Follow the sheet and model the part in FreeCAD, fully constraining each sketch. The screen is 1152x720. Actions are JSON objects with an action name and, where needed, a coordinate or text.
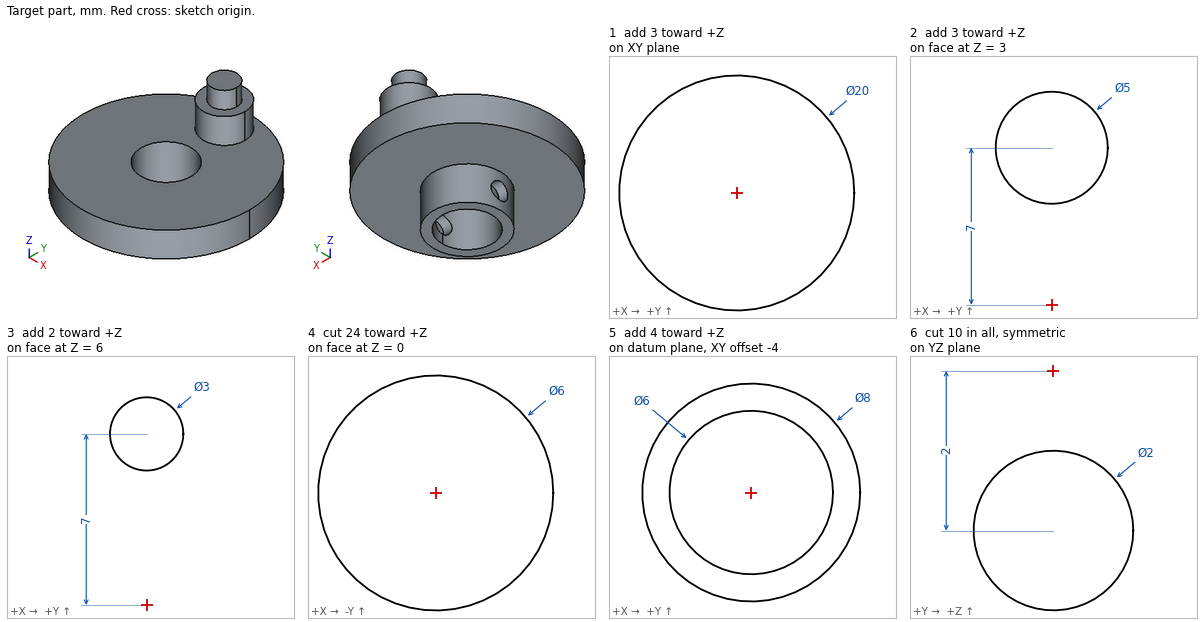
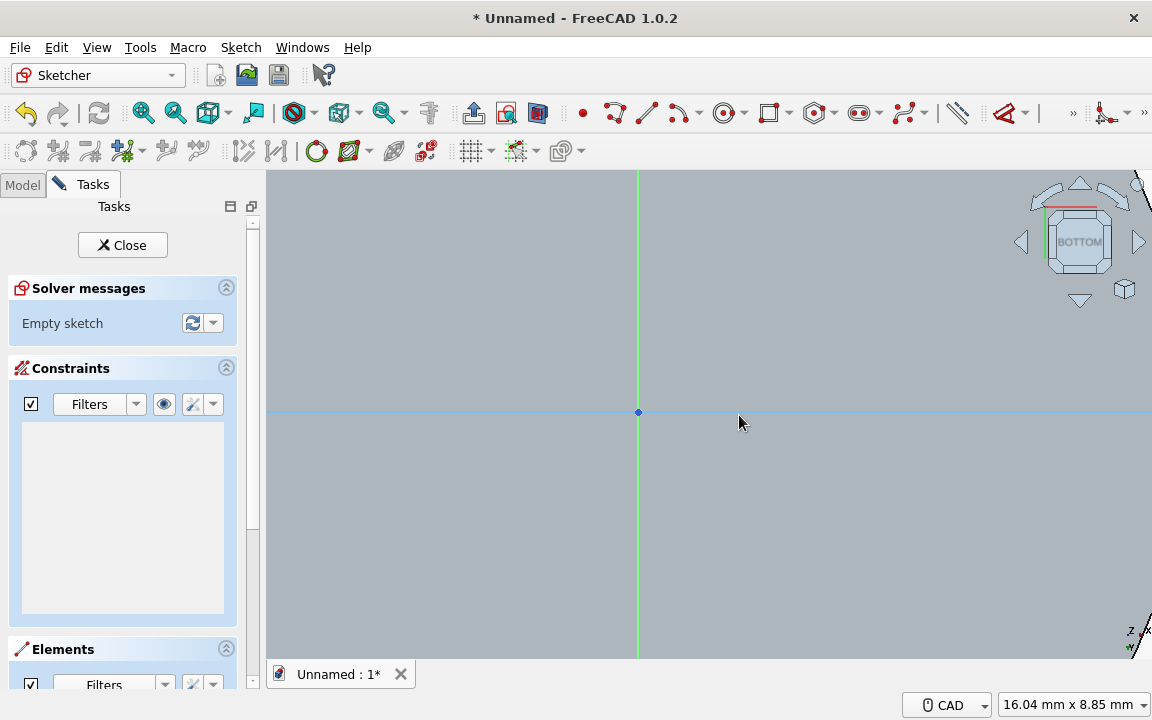
{"action": "key", "text": "g c"}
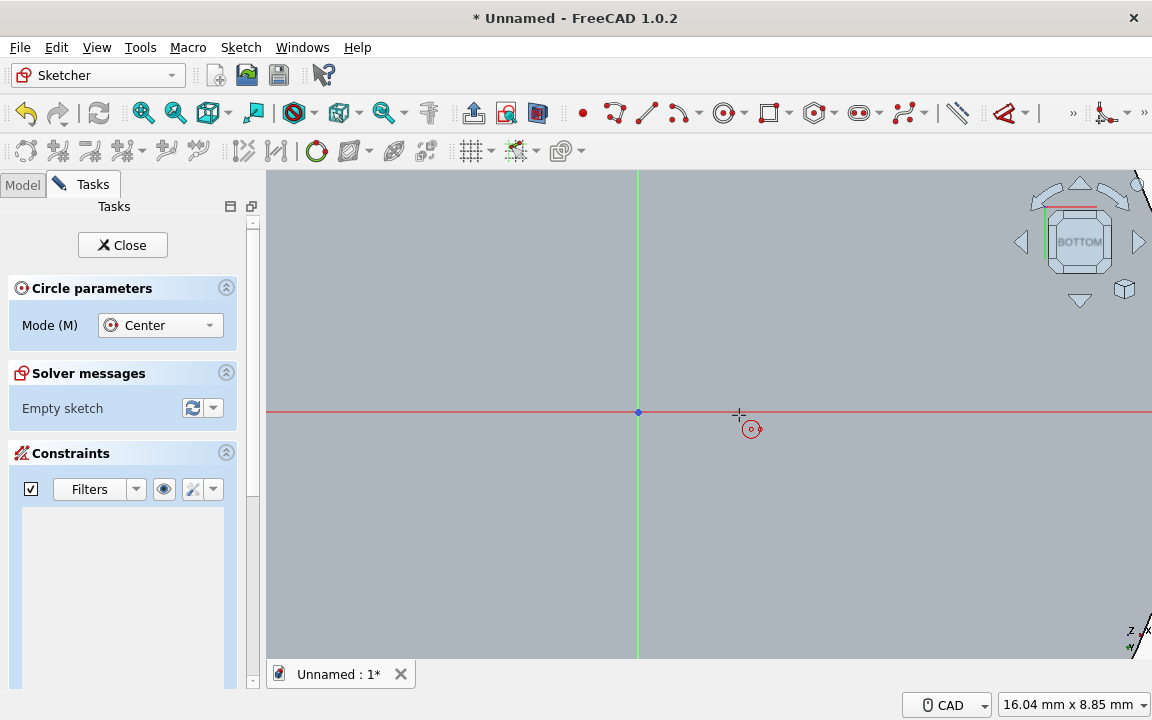
{"action": "left_click", "coordinate": [638, 412]}
{"action": "left_click", "coordinate": [755, 295]}
{"action": "key", "text": "Escape"}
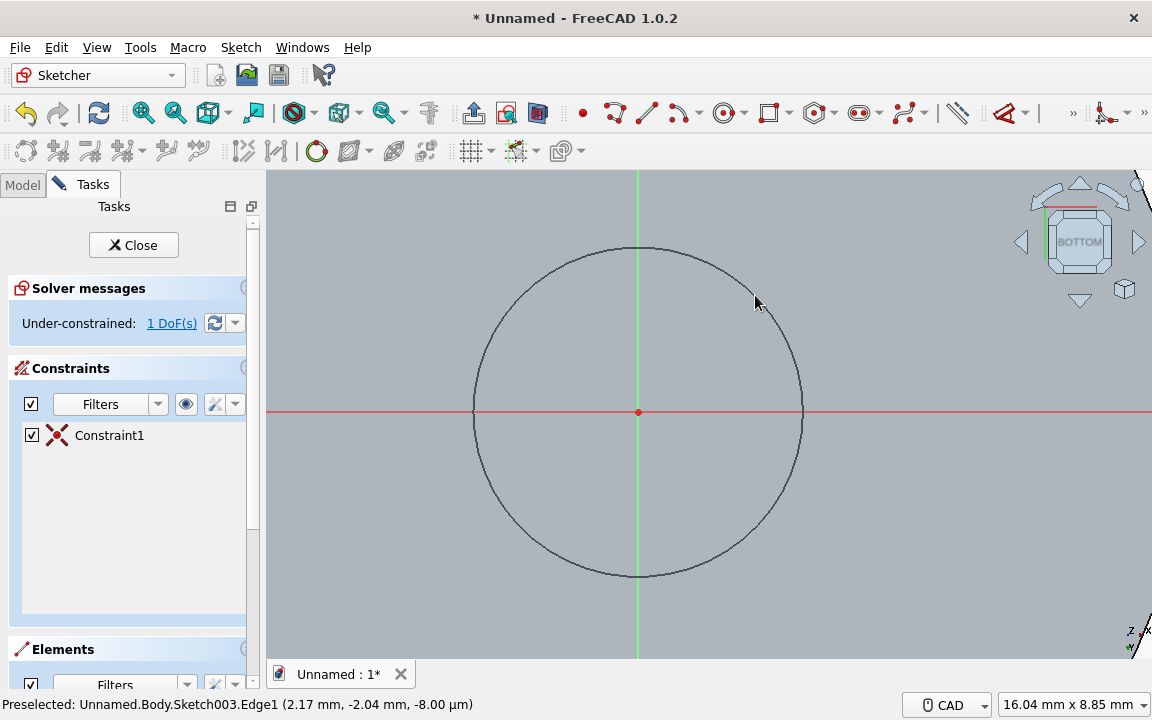
{"action": "left_click", "coordinate": [1004, 114]}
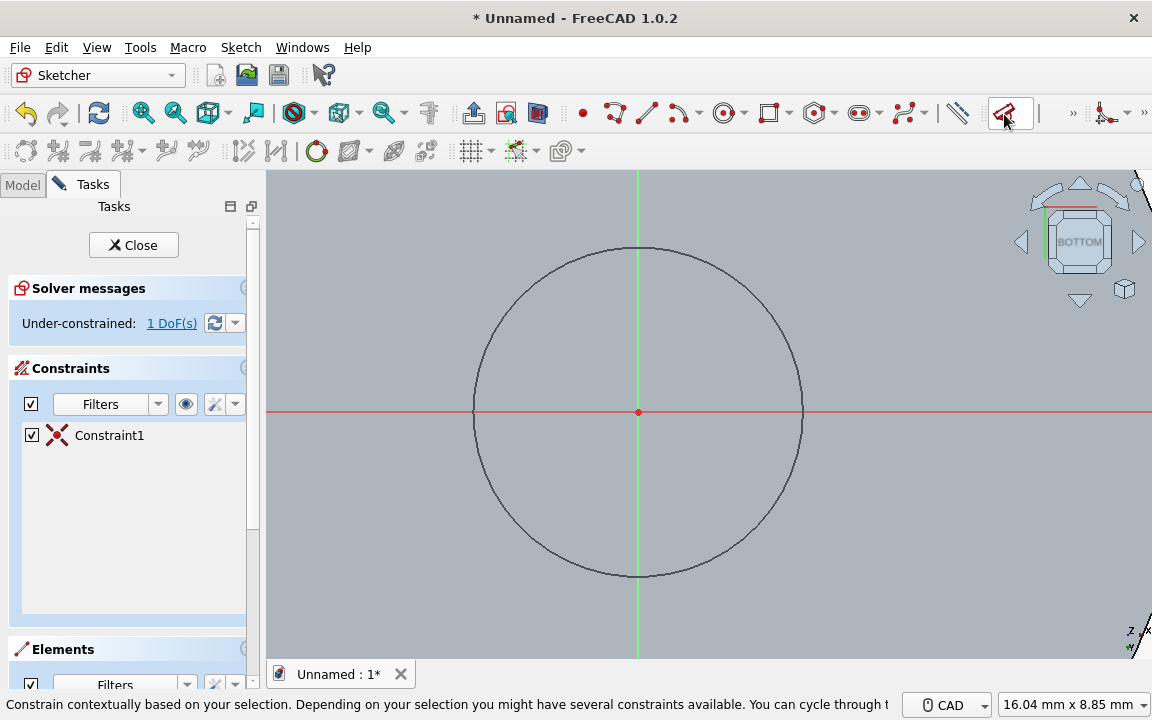
{"action": "left_click", "coordinate": [754, 295]}
{"action": "left_click", "coordinate": [776, 272]}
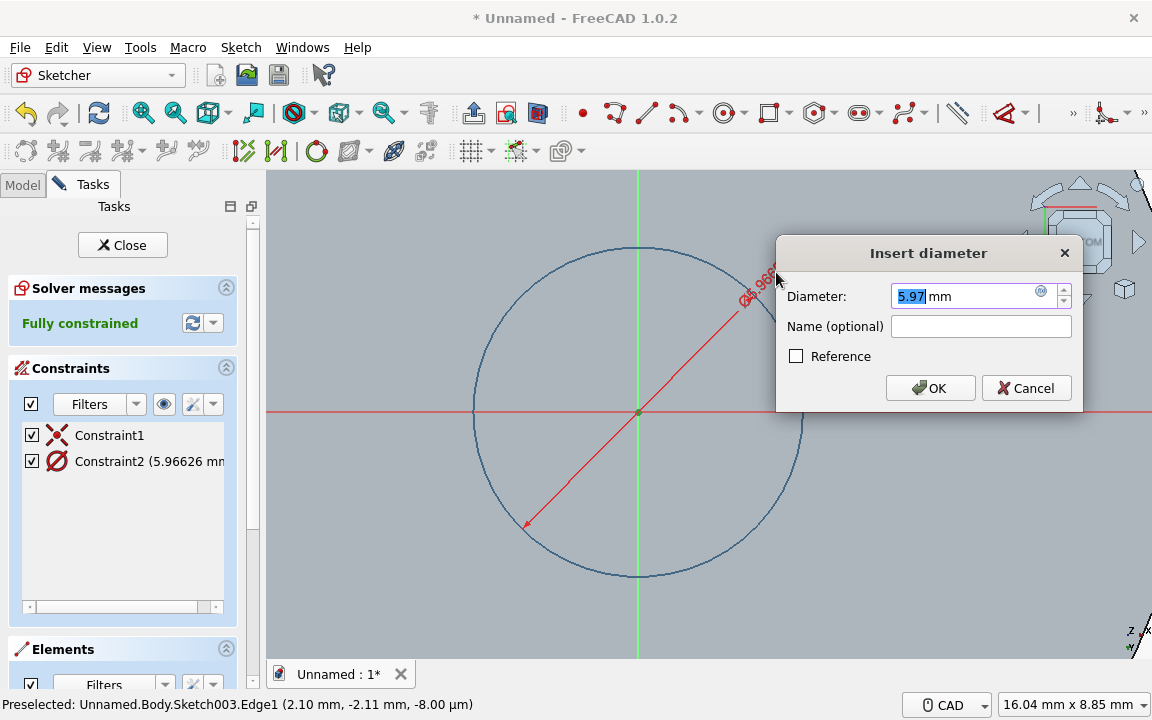
{"action": "type", "text": "6"}
{"action": "key", "text": "Return"}
{"action": "key", "text": "Escape"}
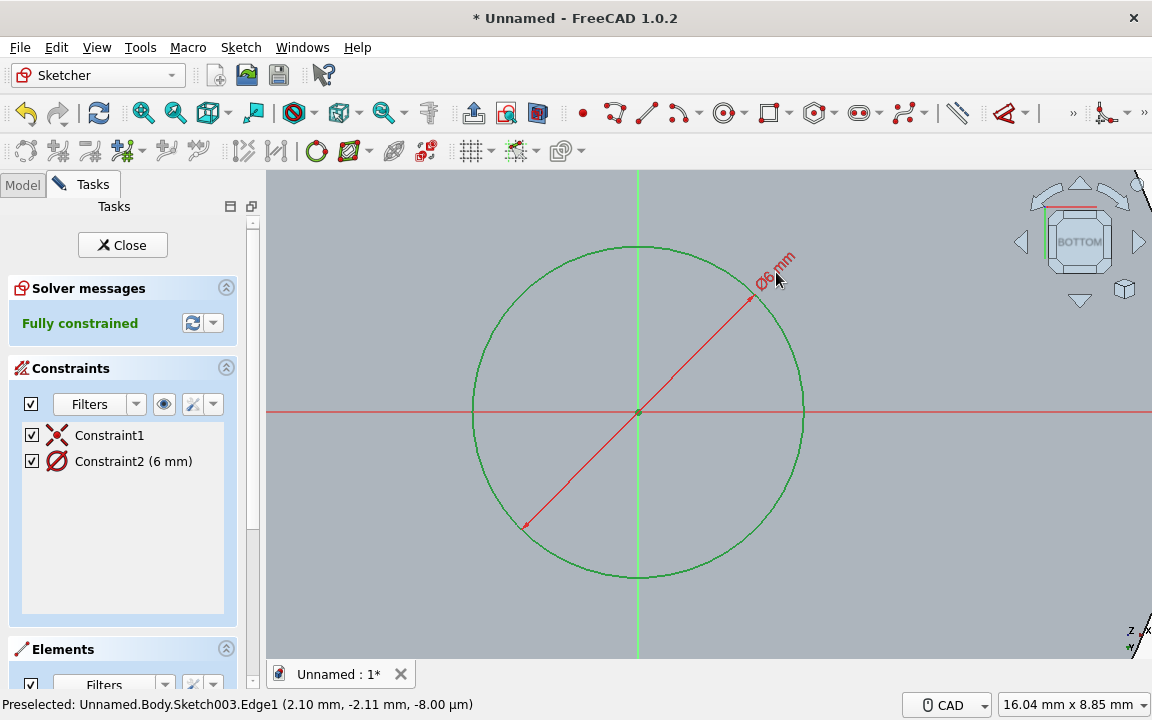
{"action": "left_click", "coordinate": [123, 245]}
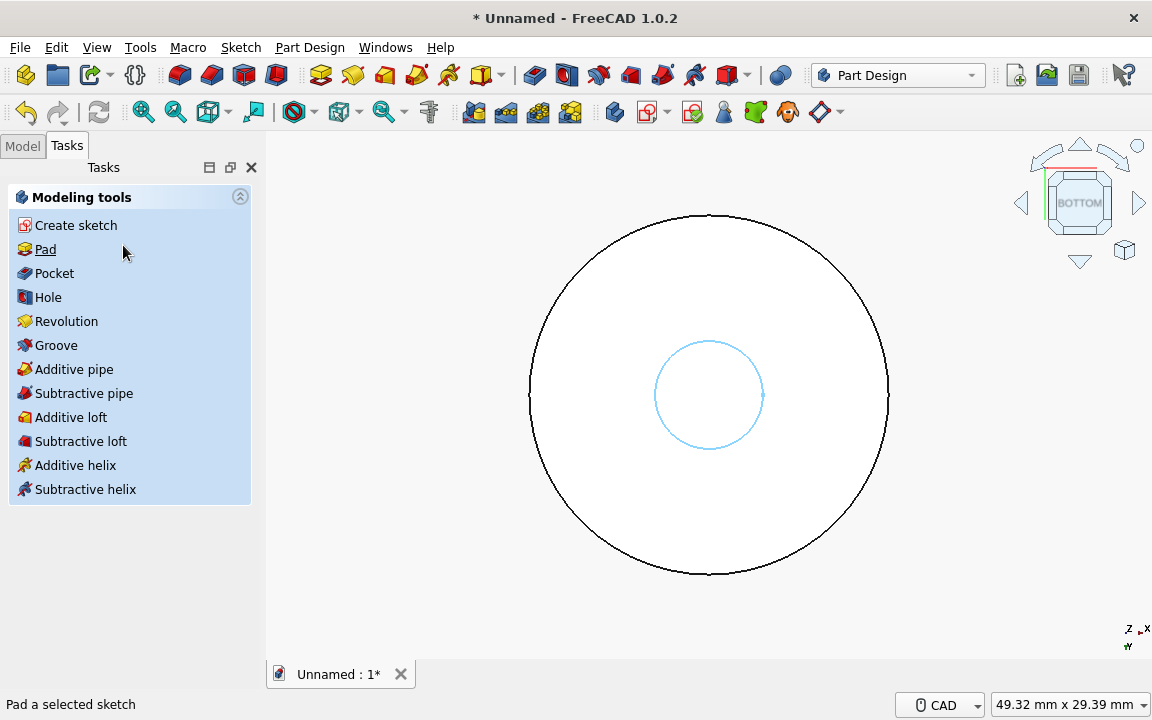
{"action": "left_click", "coordinate": [536, 76]}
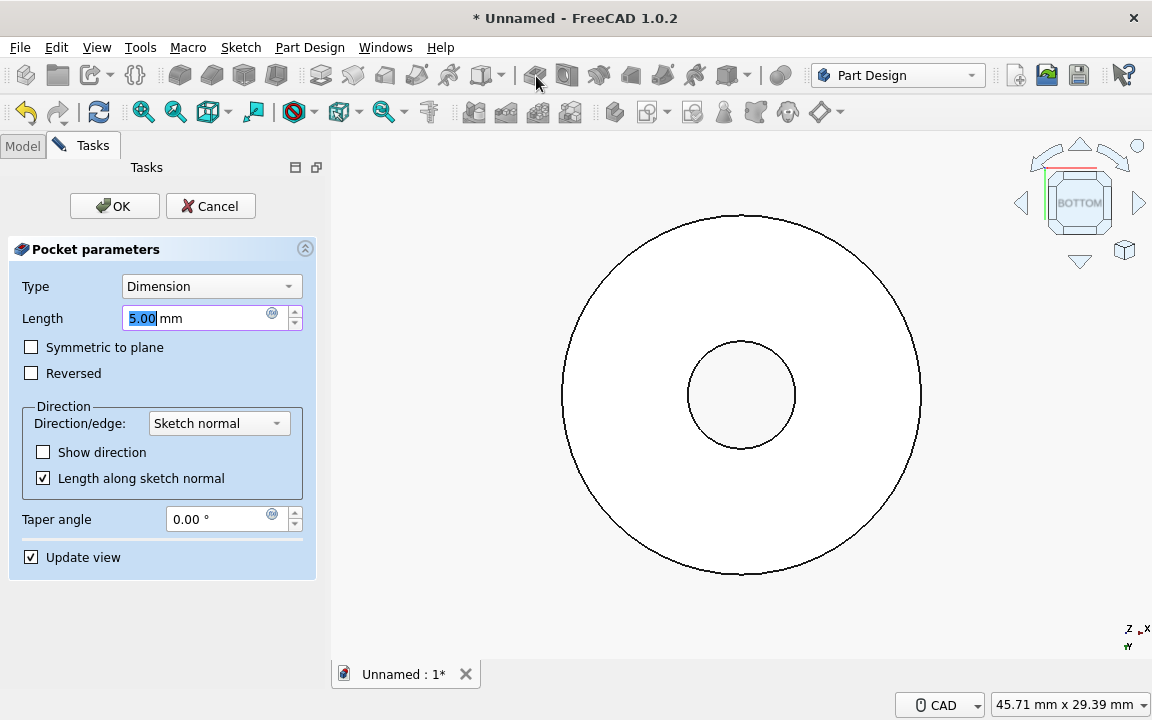
{"action": "type", "text": "24"}
{"action": "key", "text": "Tab"}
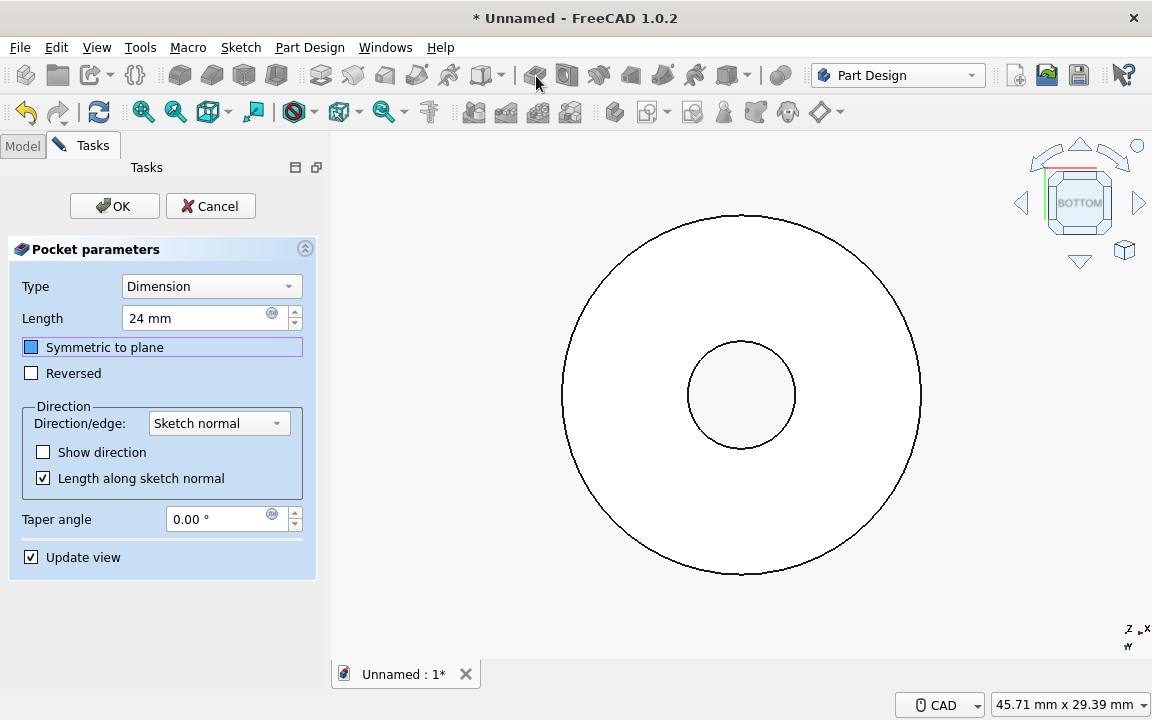
{"action": "left_click", "coordinate": [115, 206]}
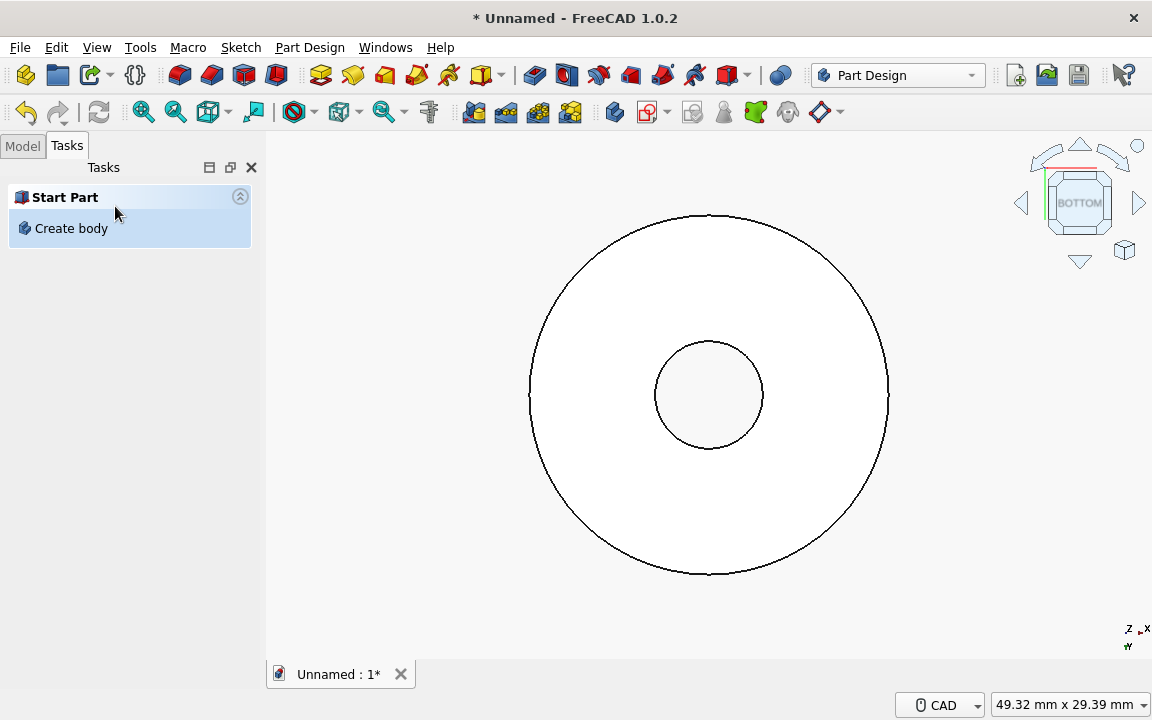
{"action": "left_click", "coordinate": [23, 145]}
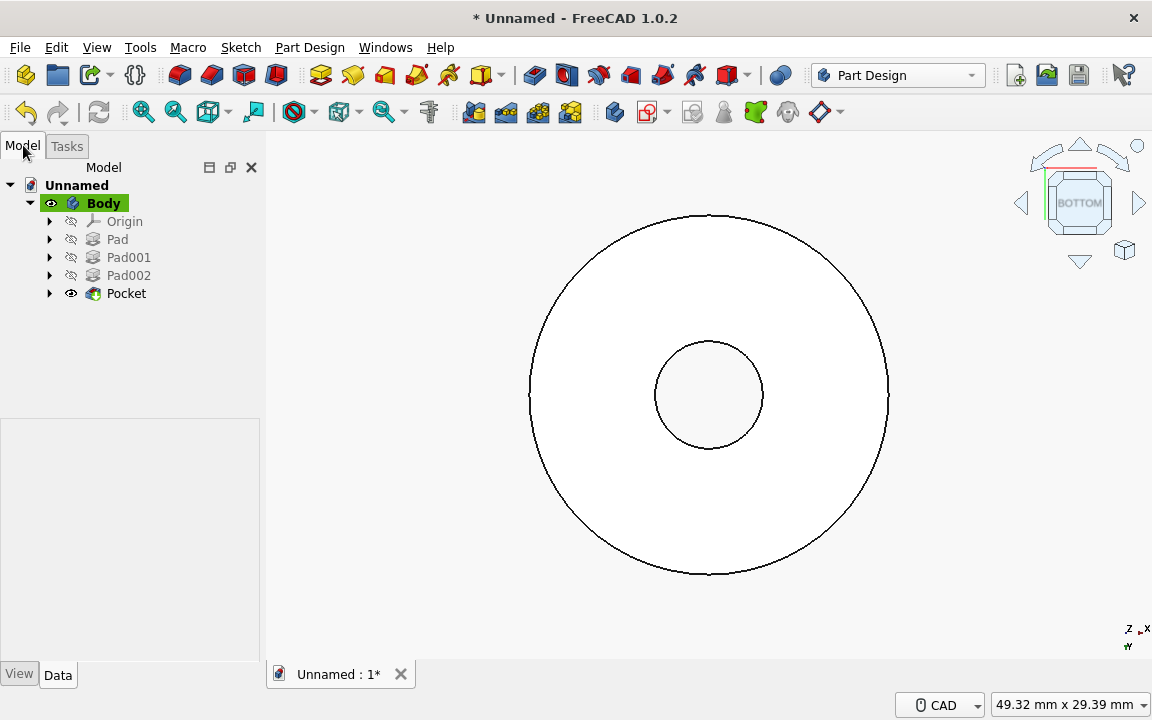
{"action": "left_click", "coordinate": [50, 221]}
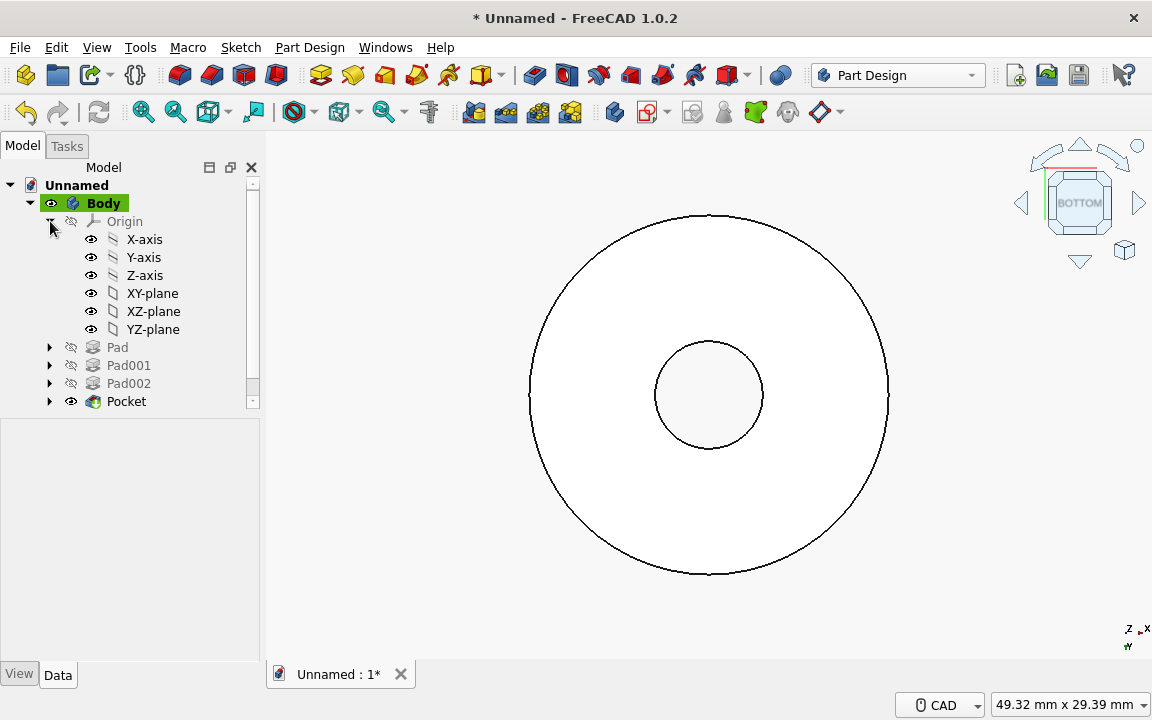
{"action": "left_click", "coordinate": [136, 293]}